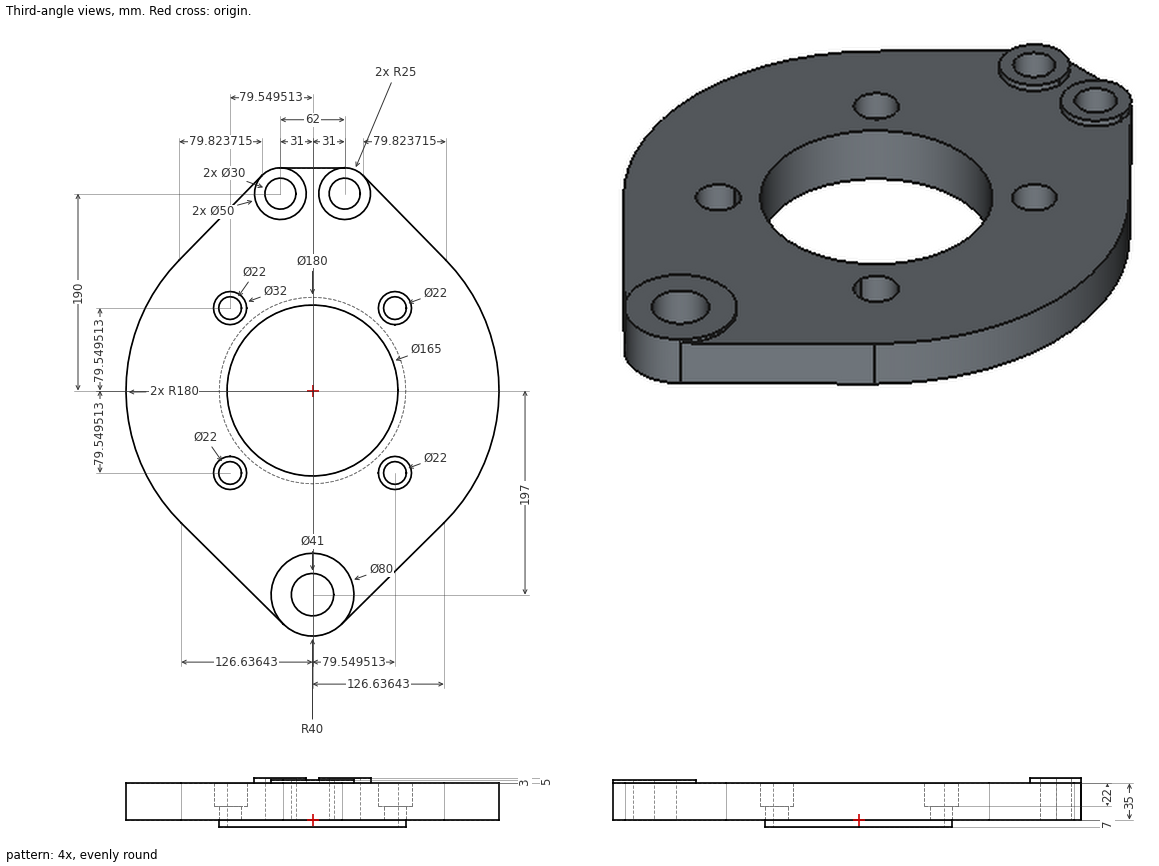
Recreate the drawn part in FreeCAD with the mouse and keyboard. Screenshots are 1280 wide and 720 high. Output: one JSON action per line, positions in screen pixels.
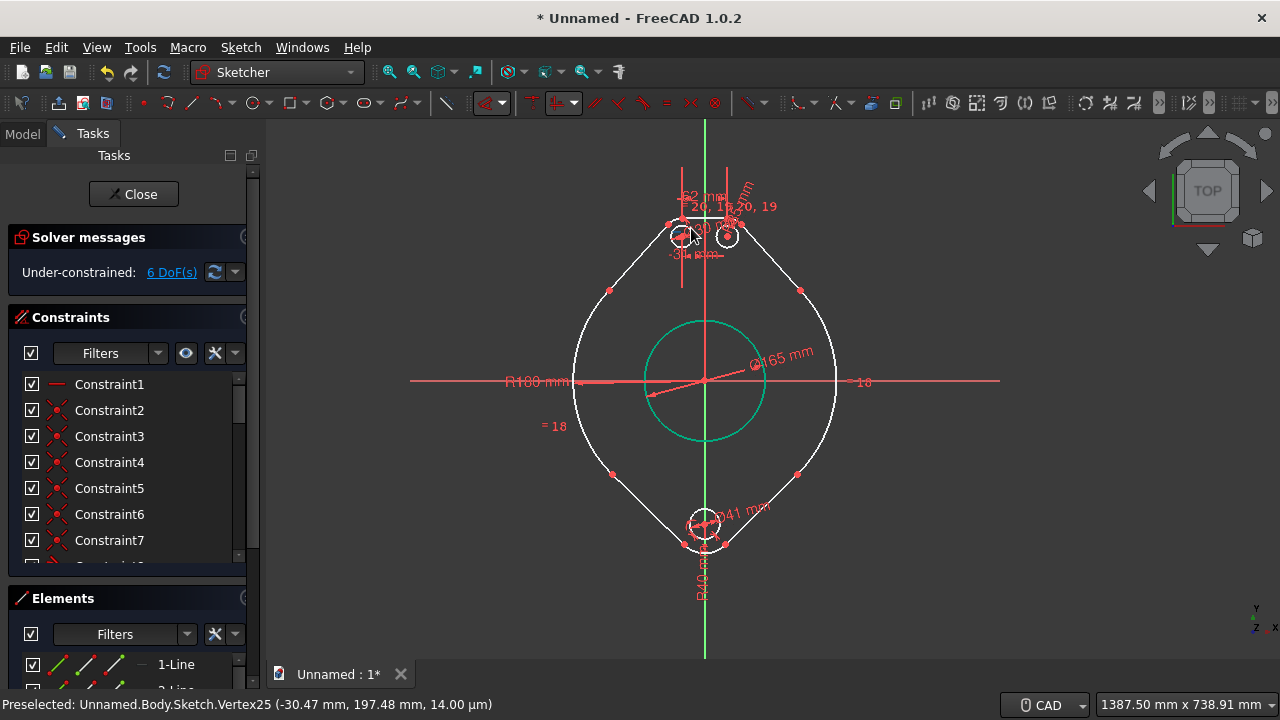
{"action": "left_click", "coordinate": [705, 524]}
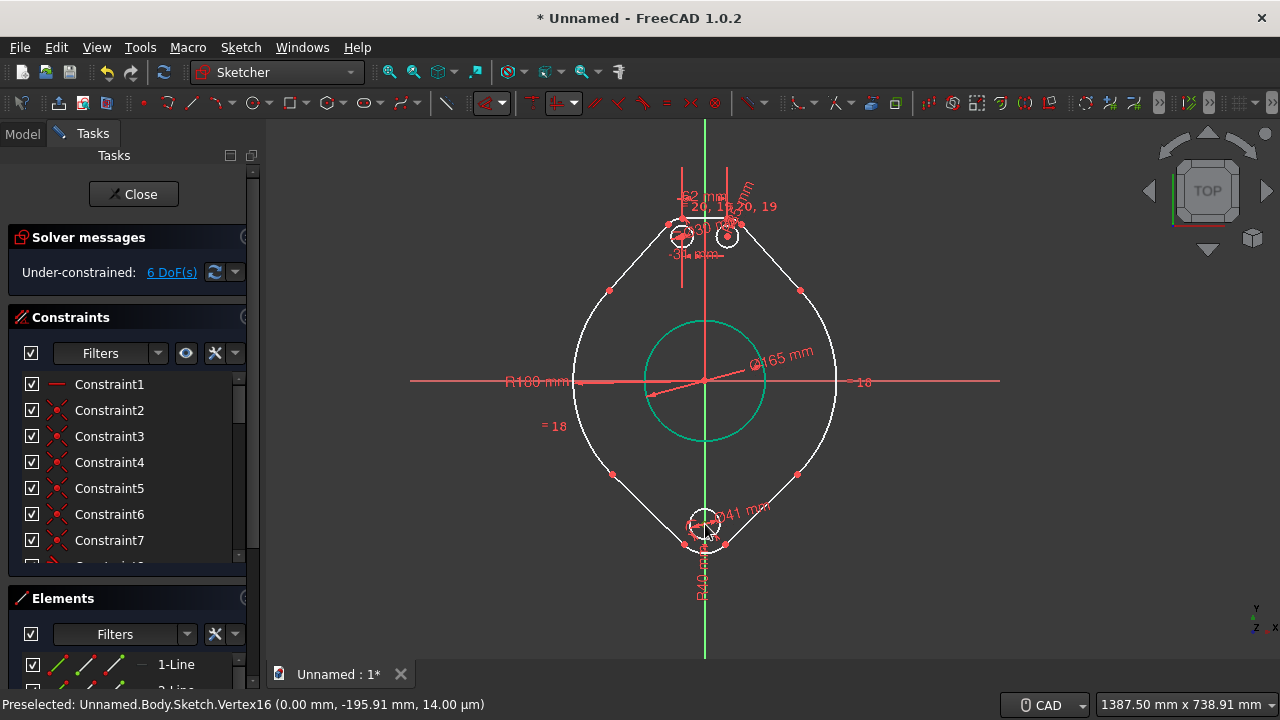
{"action": "key", "text": "i"}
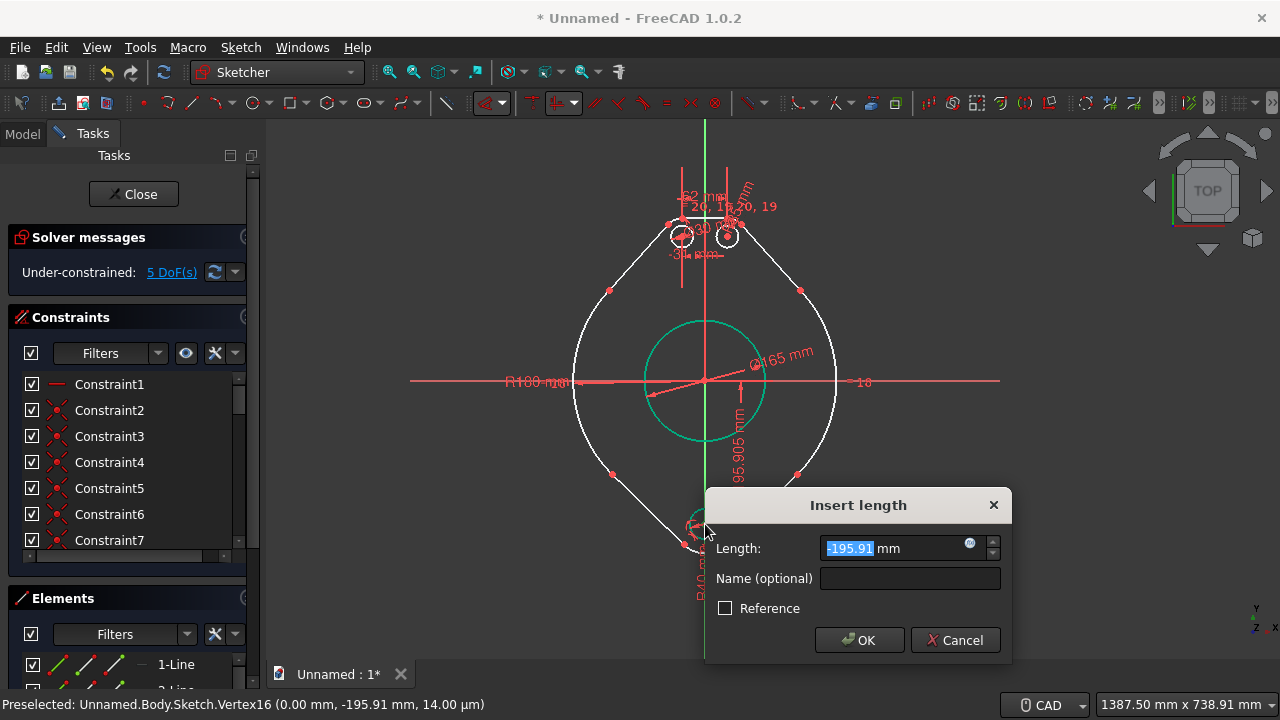
{"action": "type", "text": "-197"}
{"action": "key", "text": "Return"}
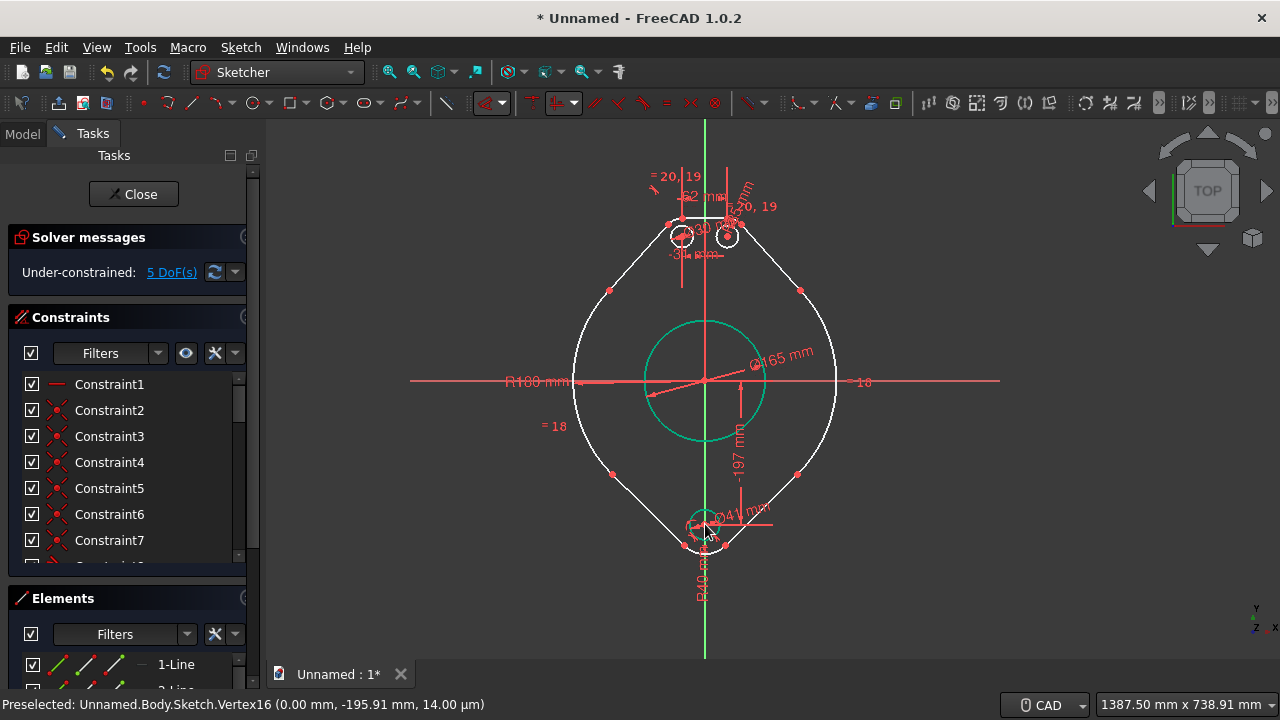
{"action": "left_click", "coordinate": [682, 237]}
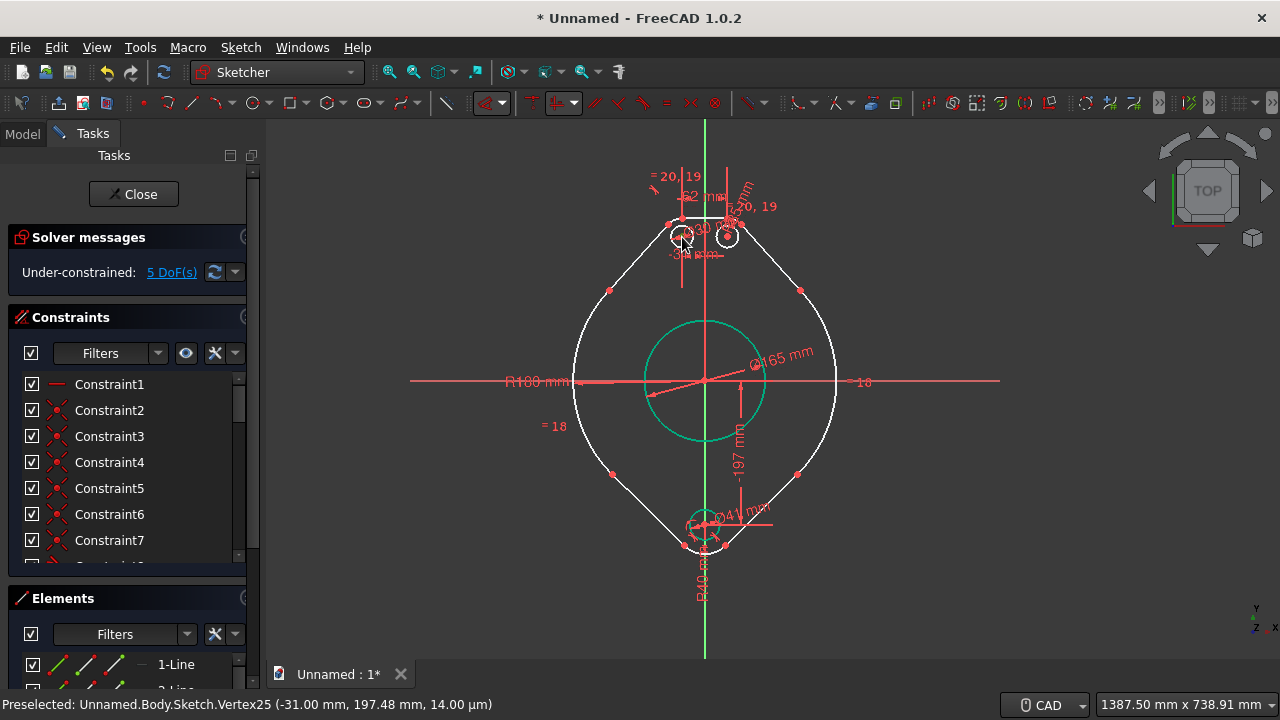
{"action": "key", "text": "i"}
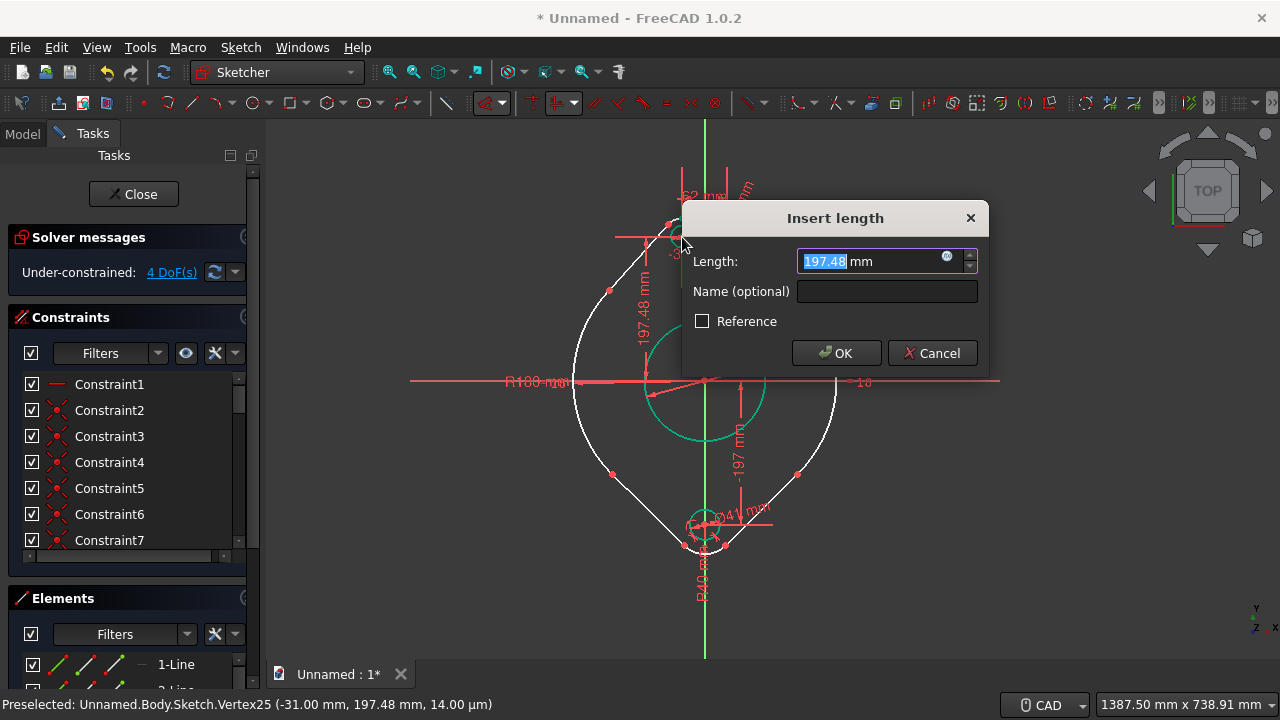
{"action": "type", "text": "190"}
{"action": "key", "text": "Return"}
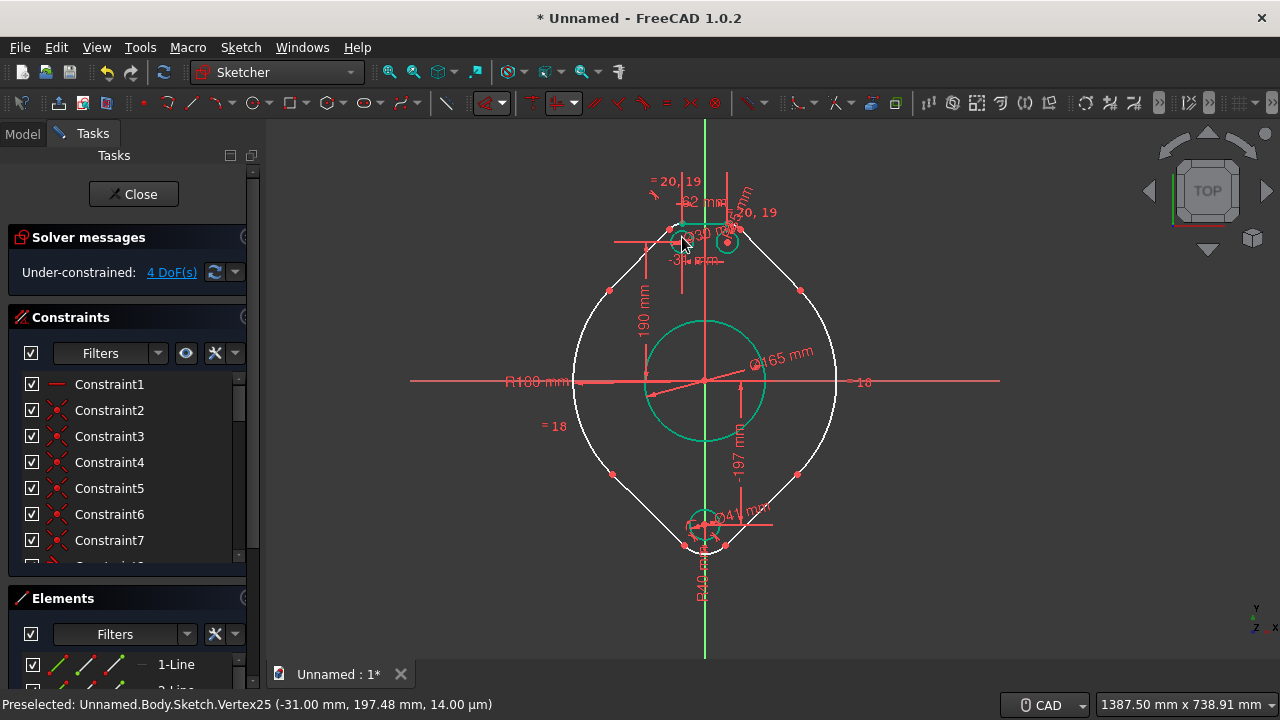
{"action": "left_click", "coordinate": [613, 475]}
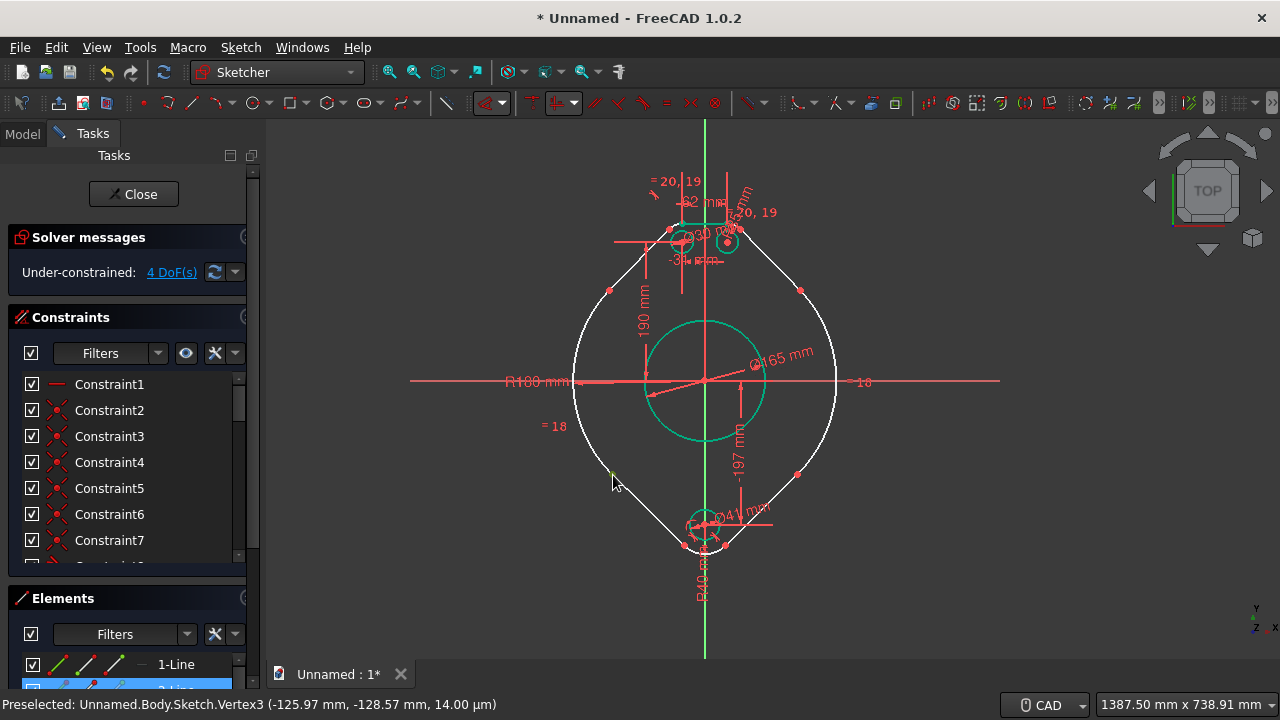
{"action": "key", "text": "l"}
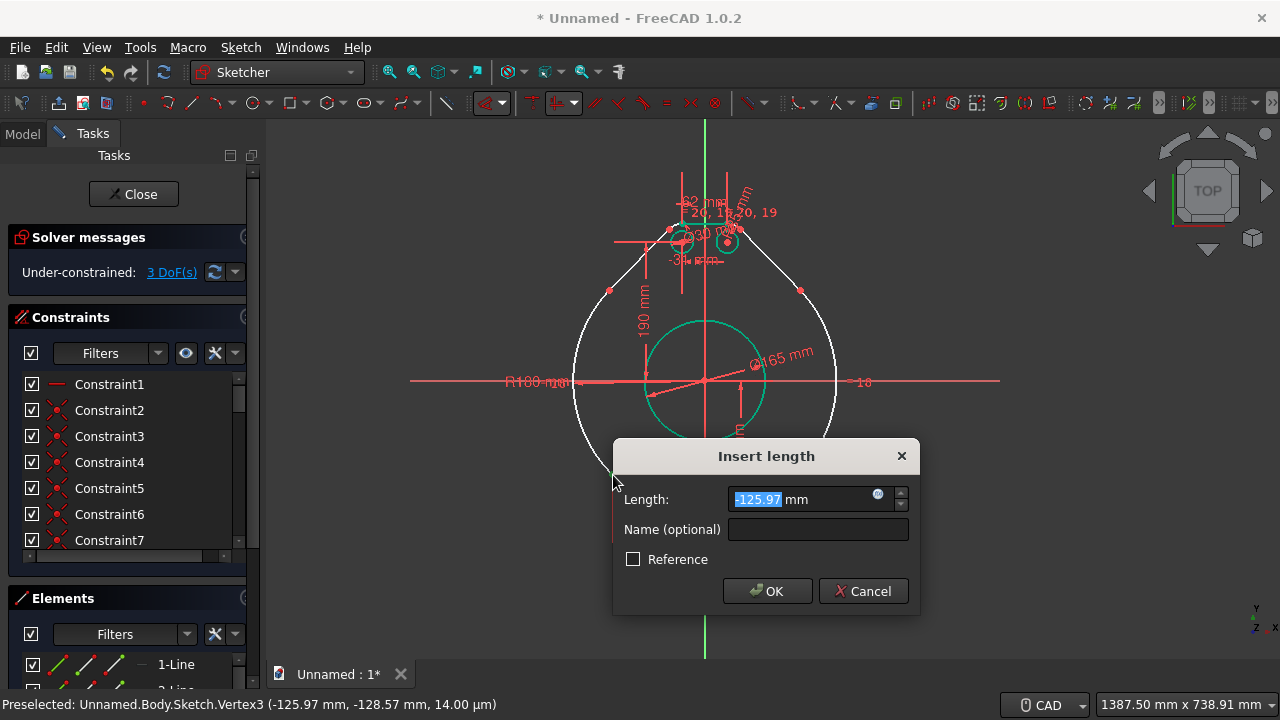
{"action": "type", "text": "-126.63643"}
{"action": "key", "text": "Return"}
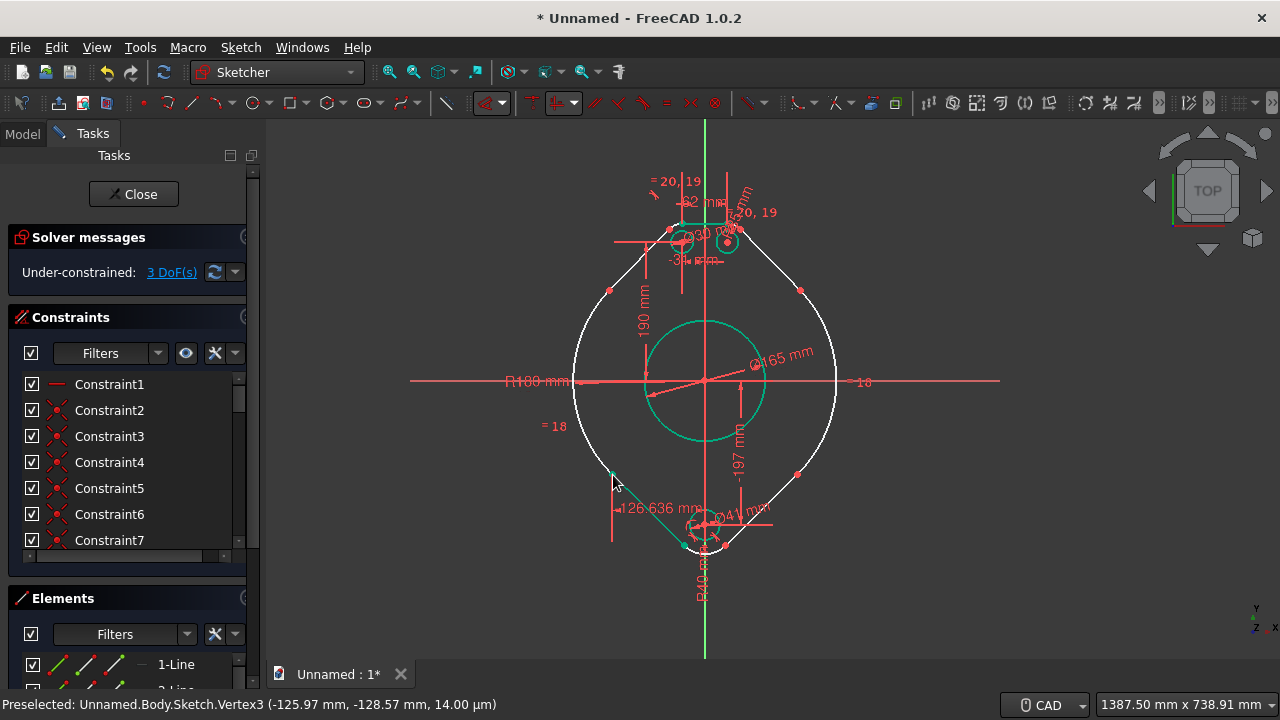
{"action": "left_click", "coordinate": [798, 474]}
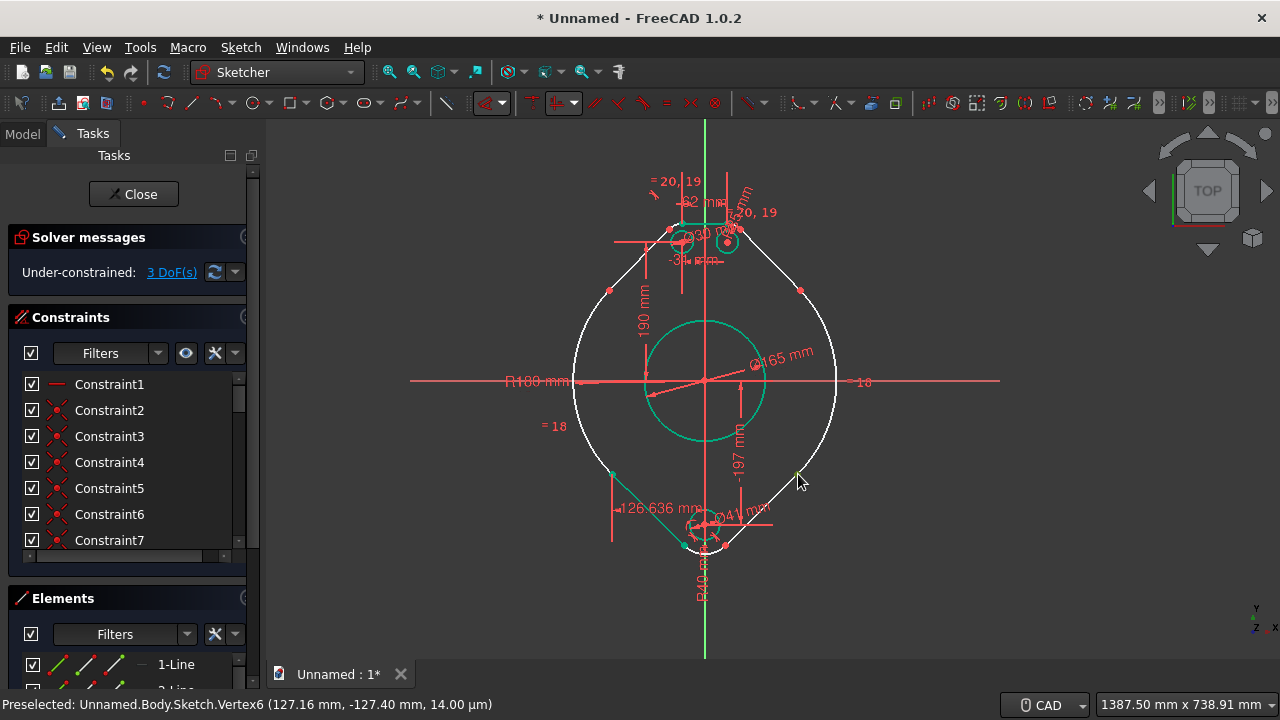
{"action": "key", "text": "l"}